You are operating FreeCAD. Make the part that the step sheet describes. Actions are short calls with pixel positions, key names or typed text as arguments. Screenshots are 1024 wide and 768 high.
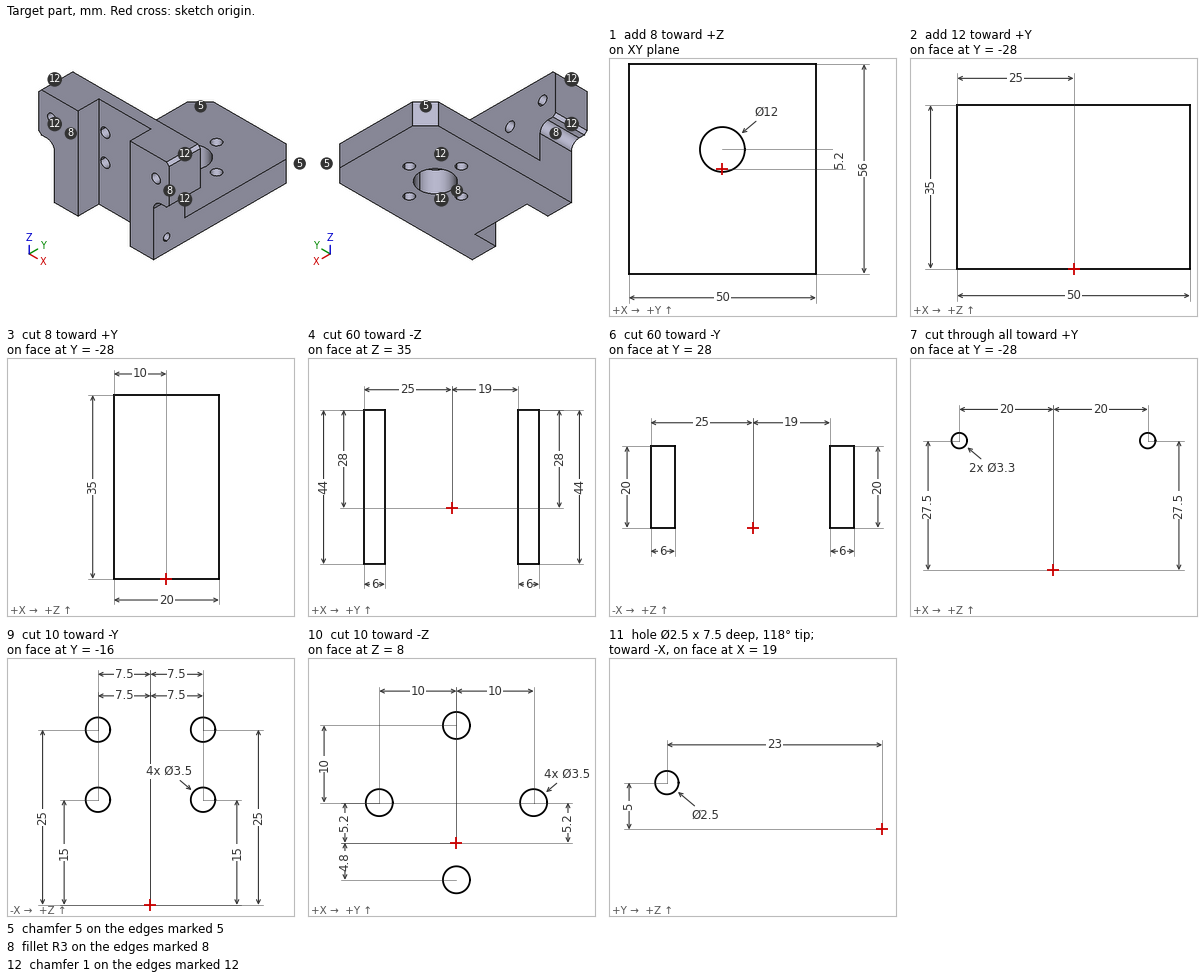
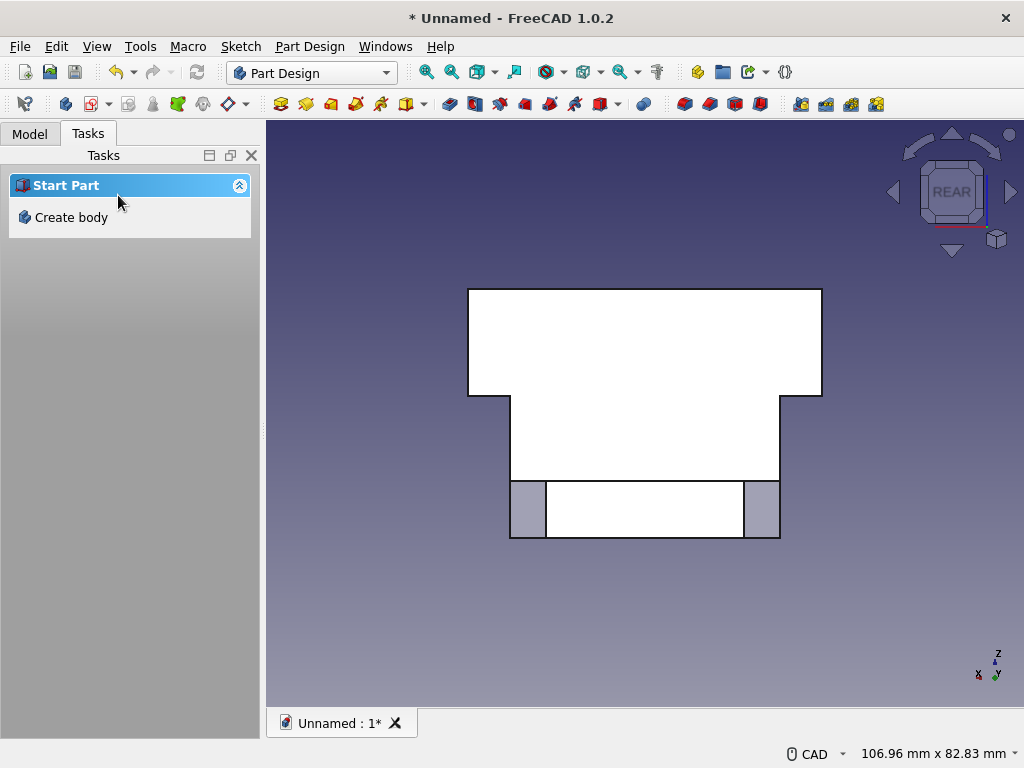
key(0)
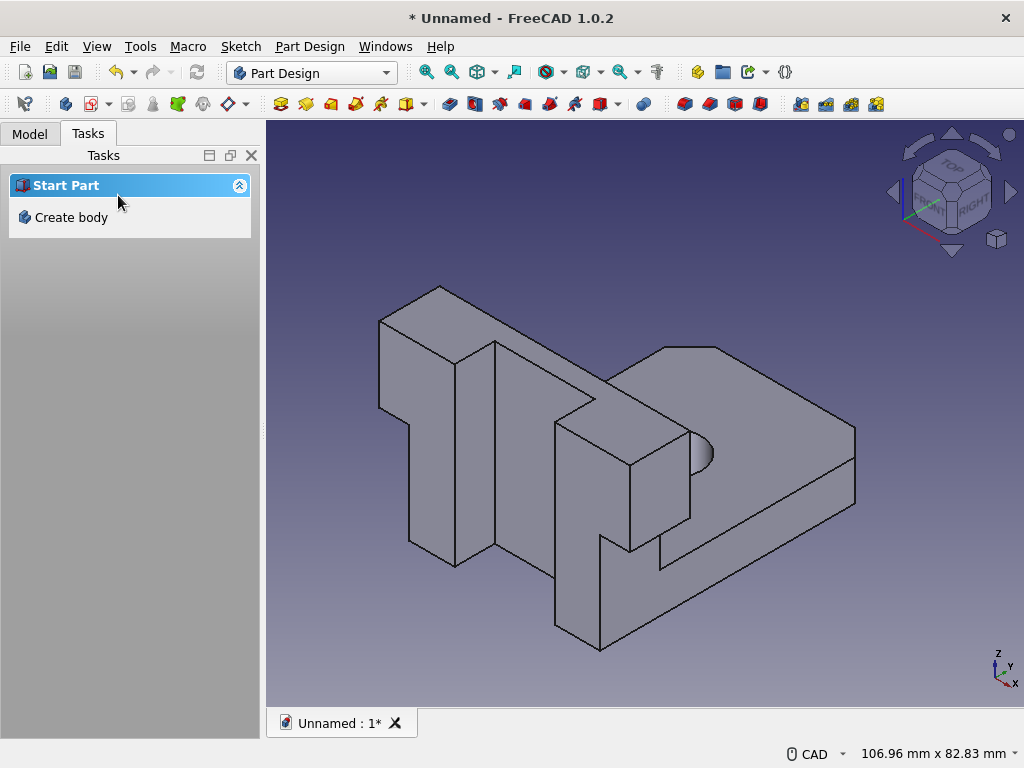
click(592, 486)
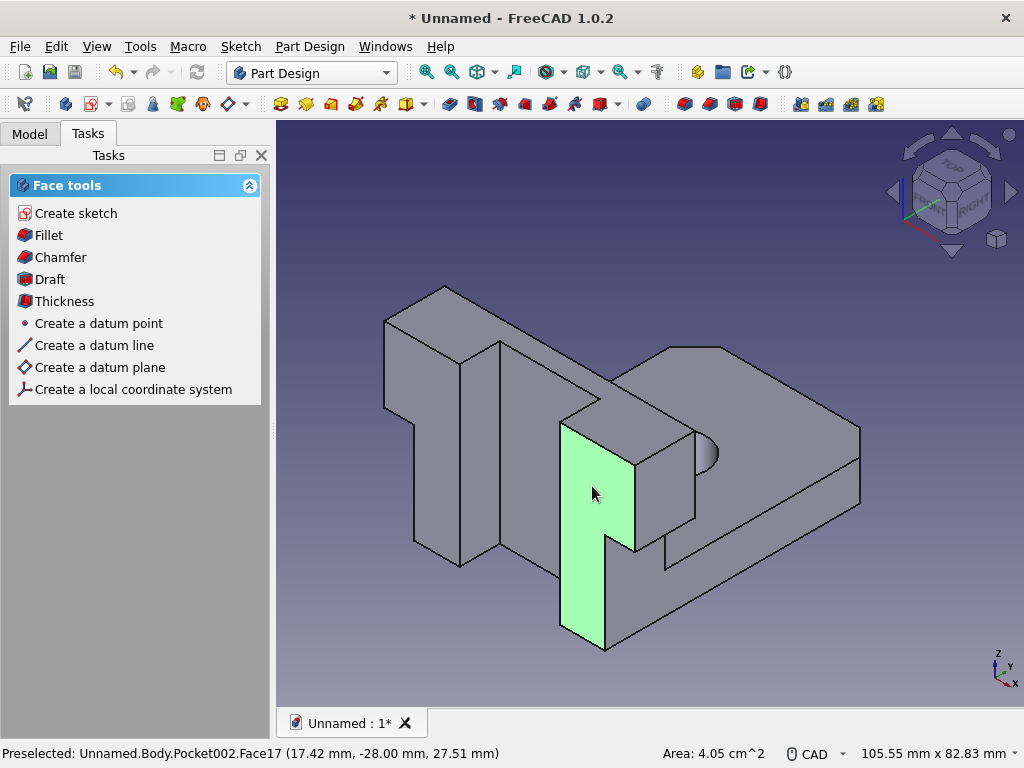
click(90, 104)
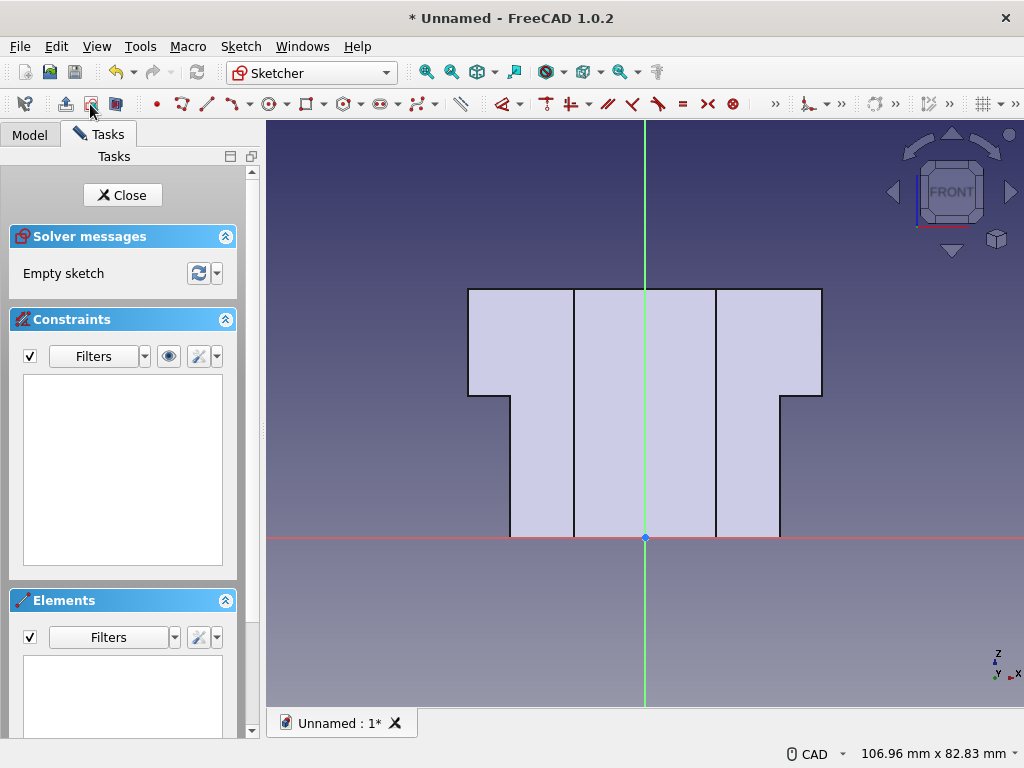
click(268, 104)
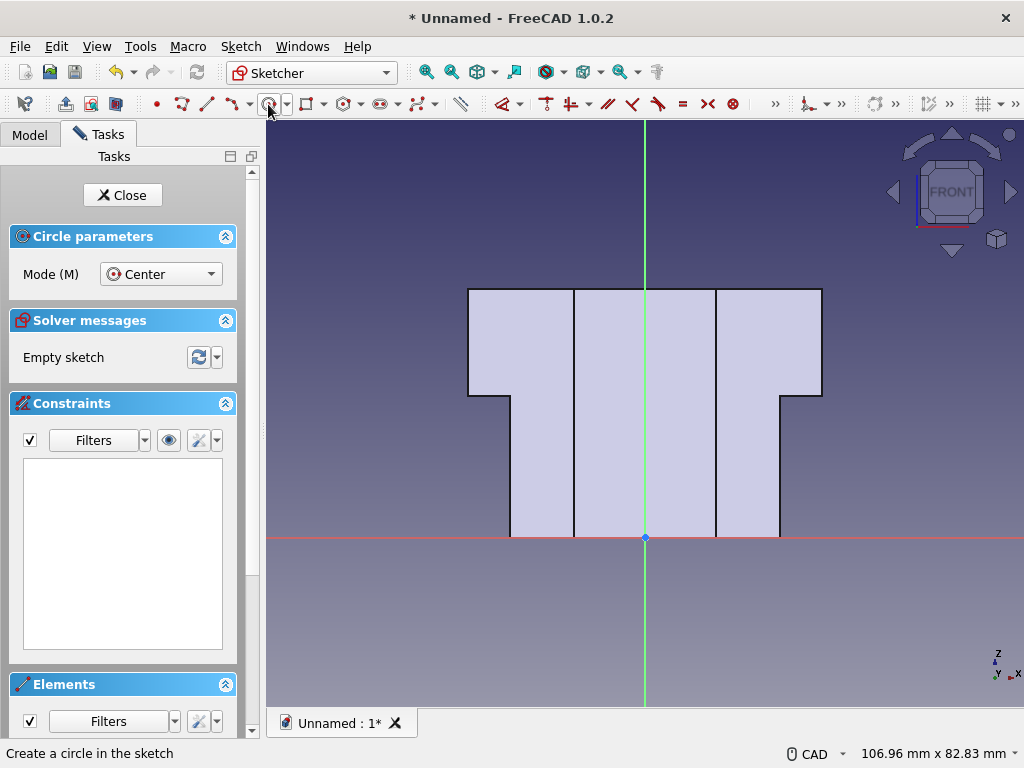
scroll(503, 343, up, 4)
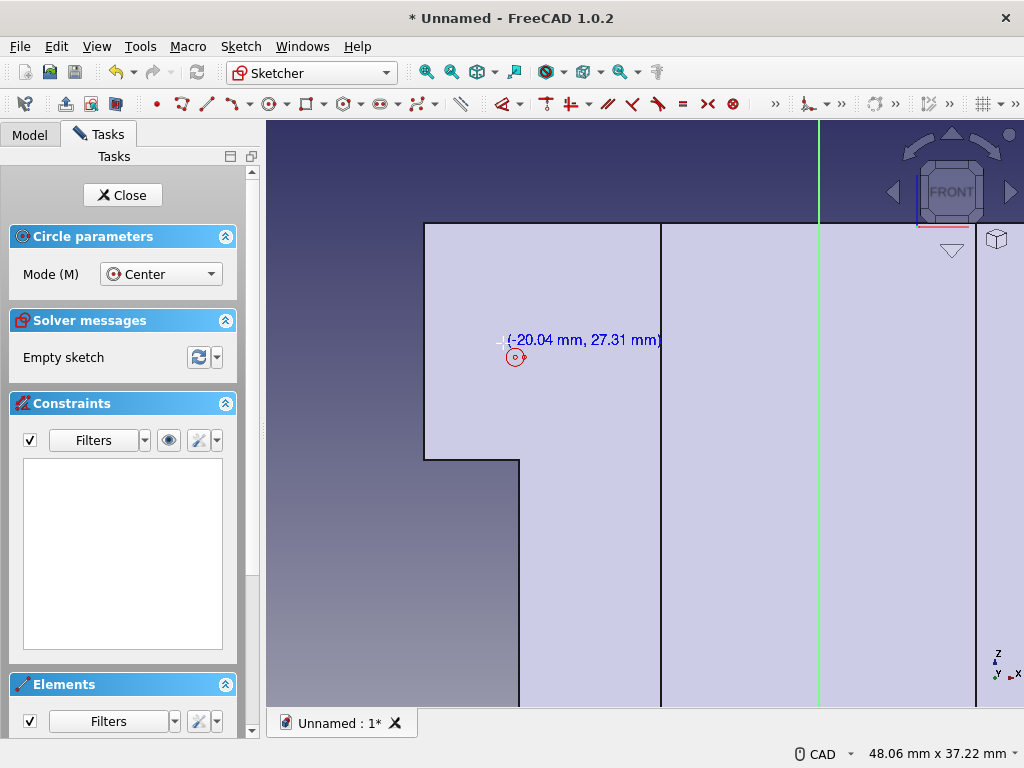
click(503, 342)
move(522, 323)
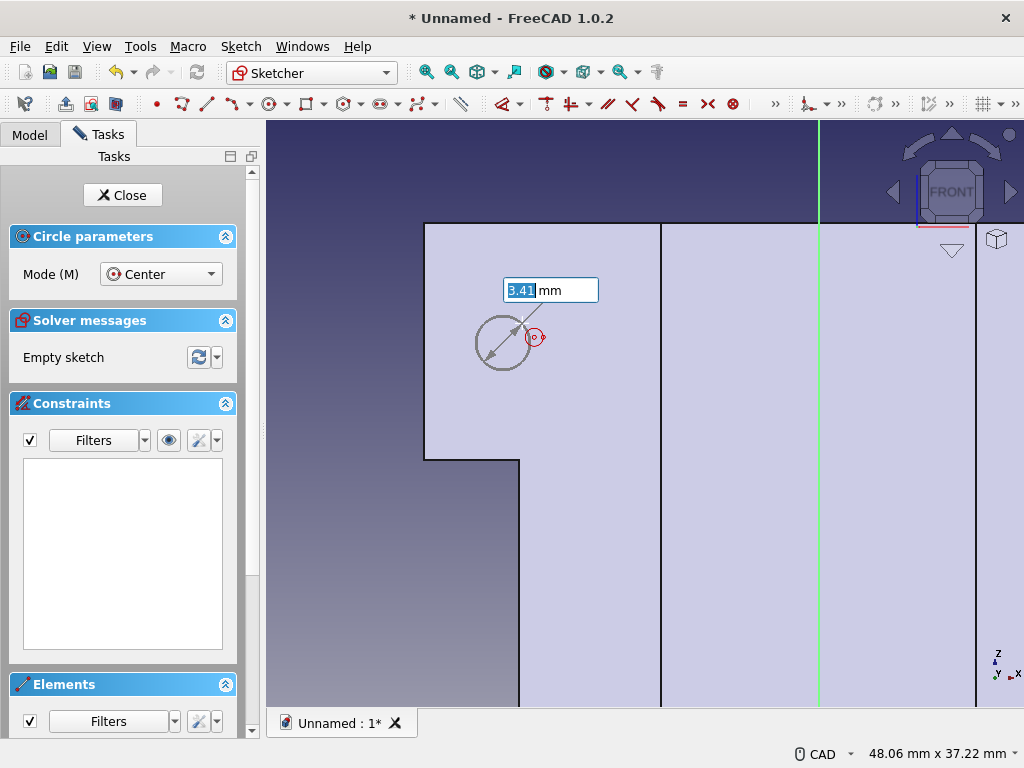
text(3.3)
key(Return)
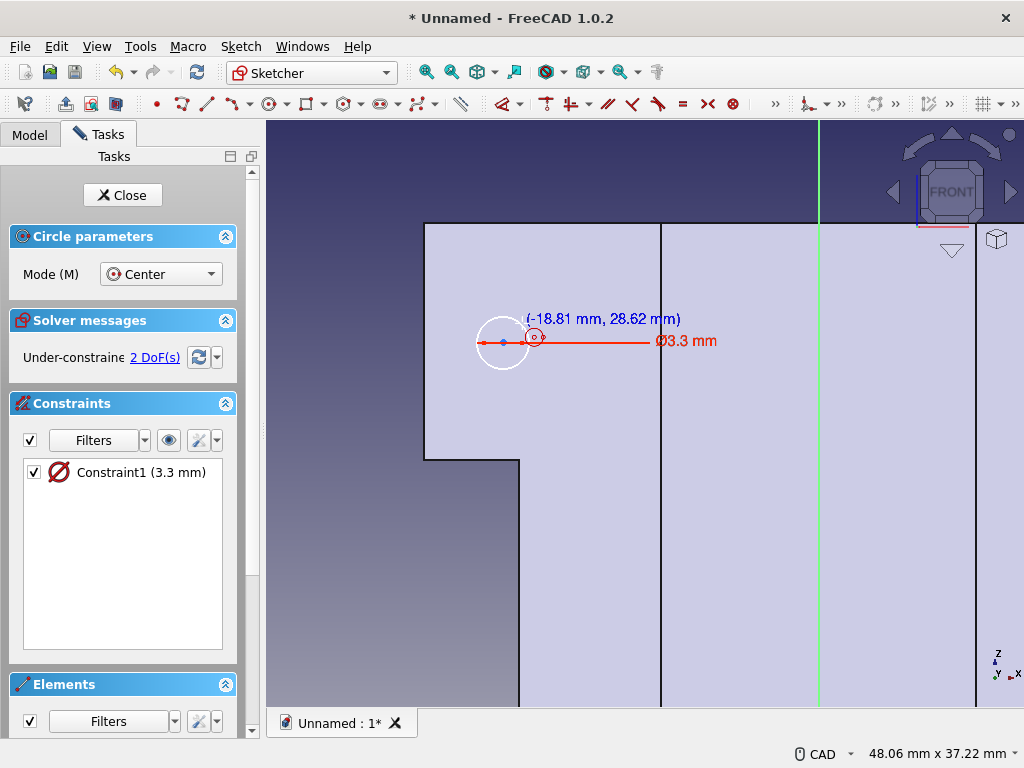
scroll(294, 253, down, 3)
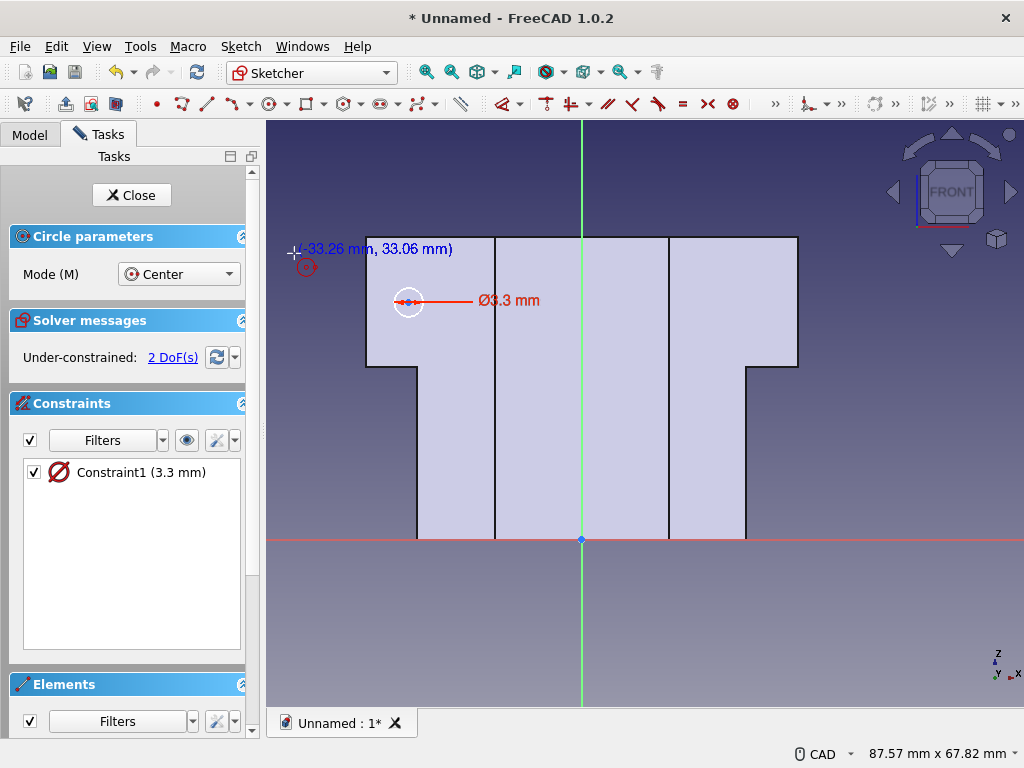
scroll(755, 302, up, 3)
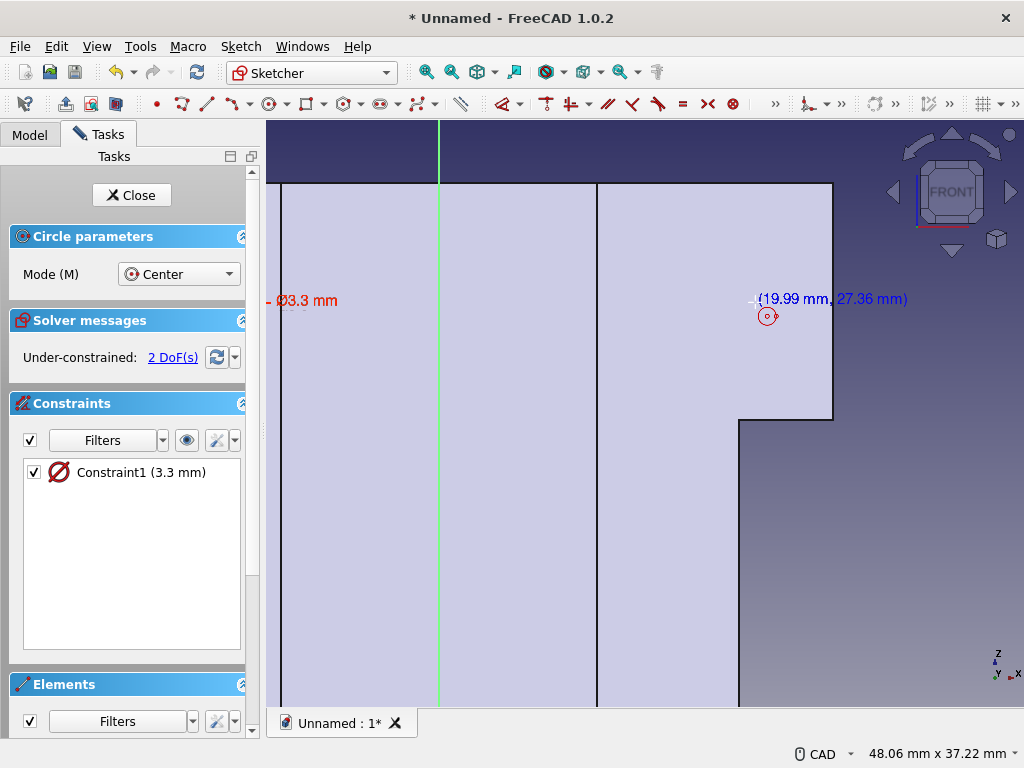
click(755, 301)
move(773, 283)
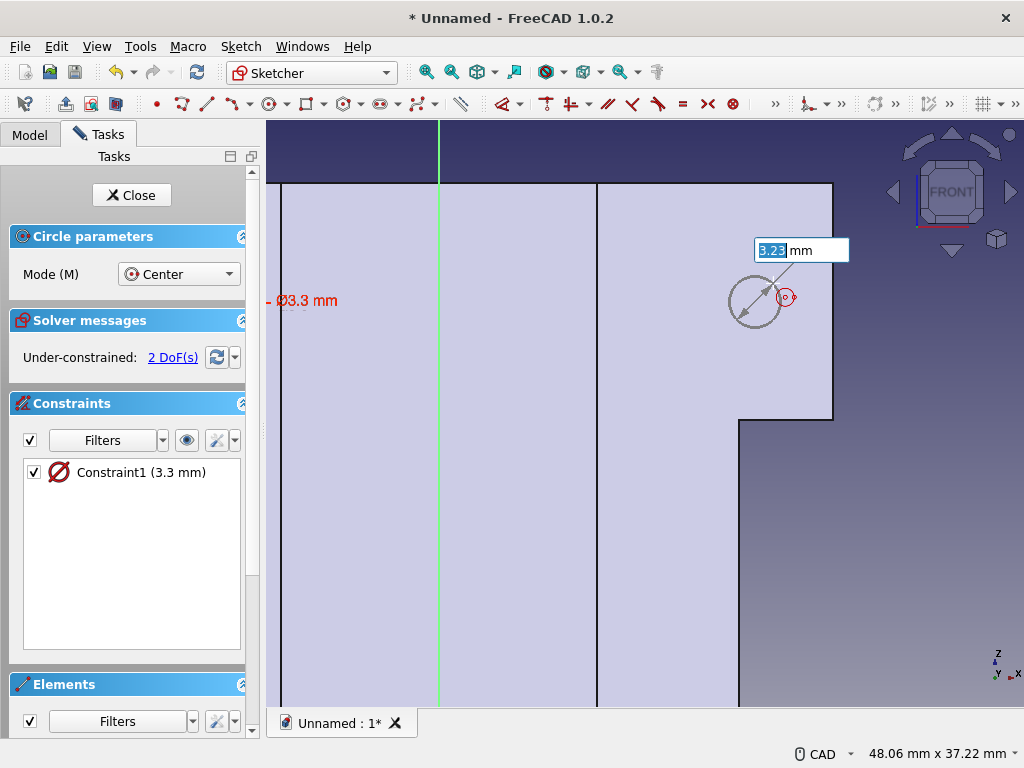
text(3.3)
key(Return)
key(Escape)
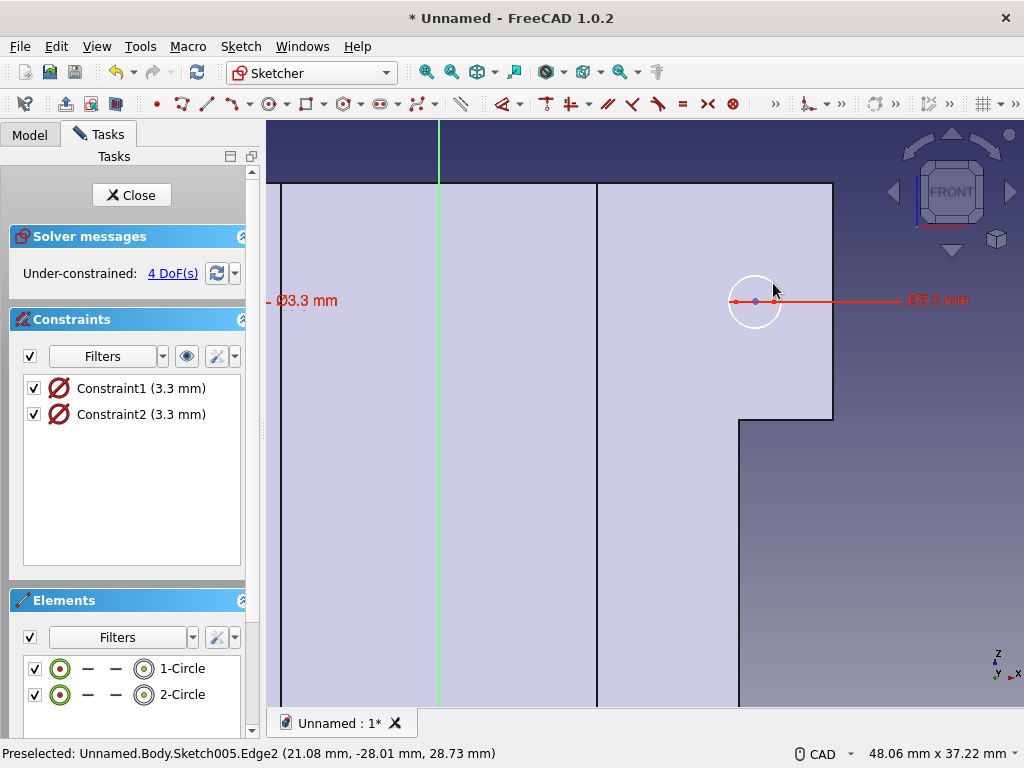
click(502, 104)